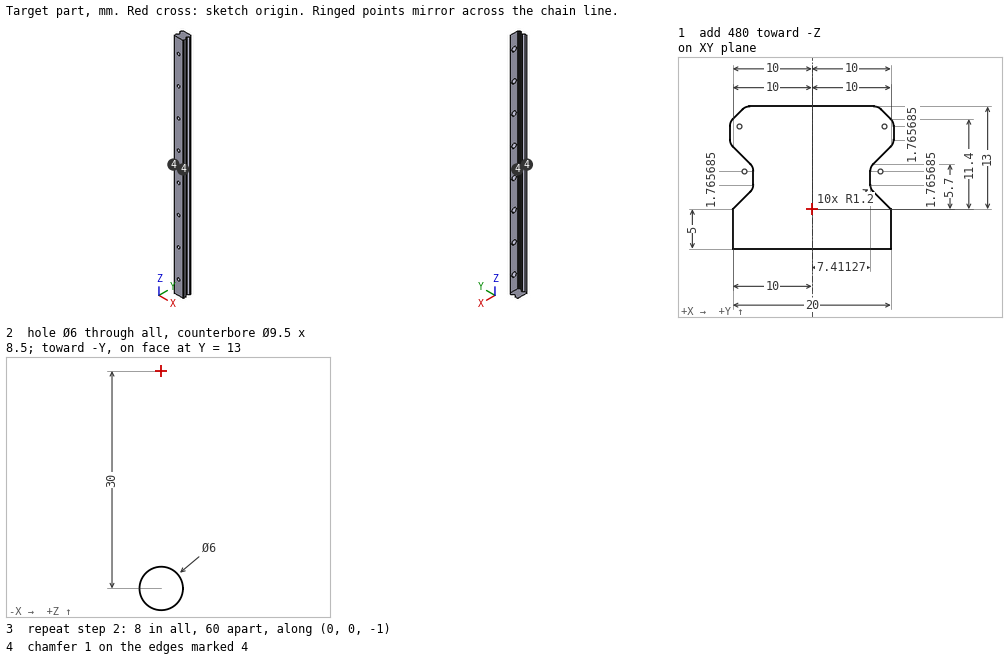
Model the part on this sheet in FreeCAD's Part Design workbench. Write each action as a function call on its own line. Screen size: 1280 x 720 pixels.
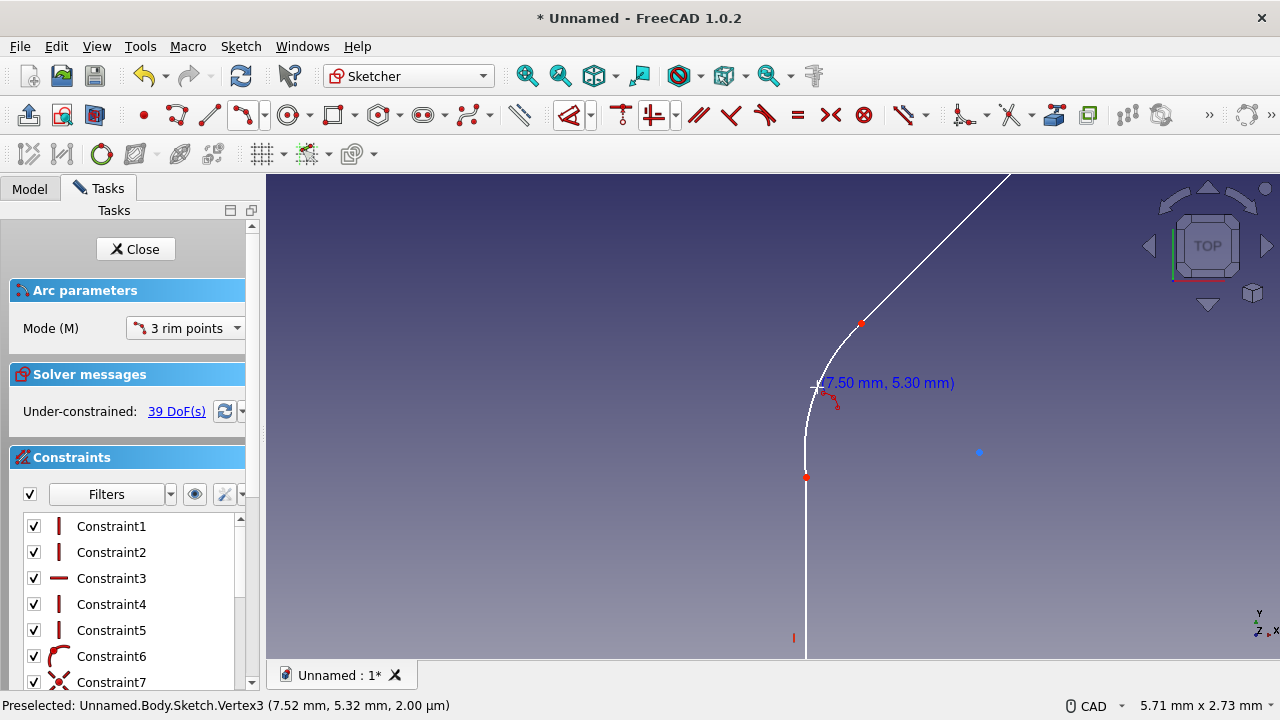
scroll(826, 396, down, 12)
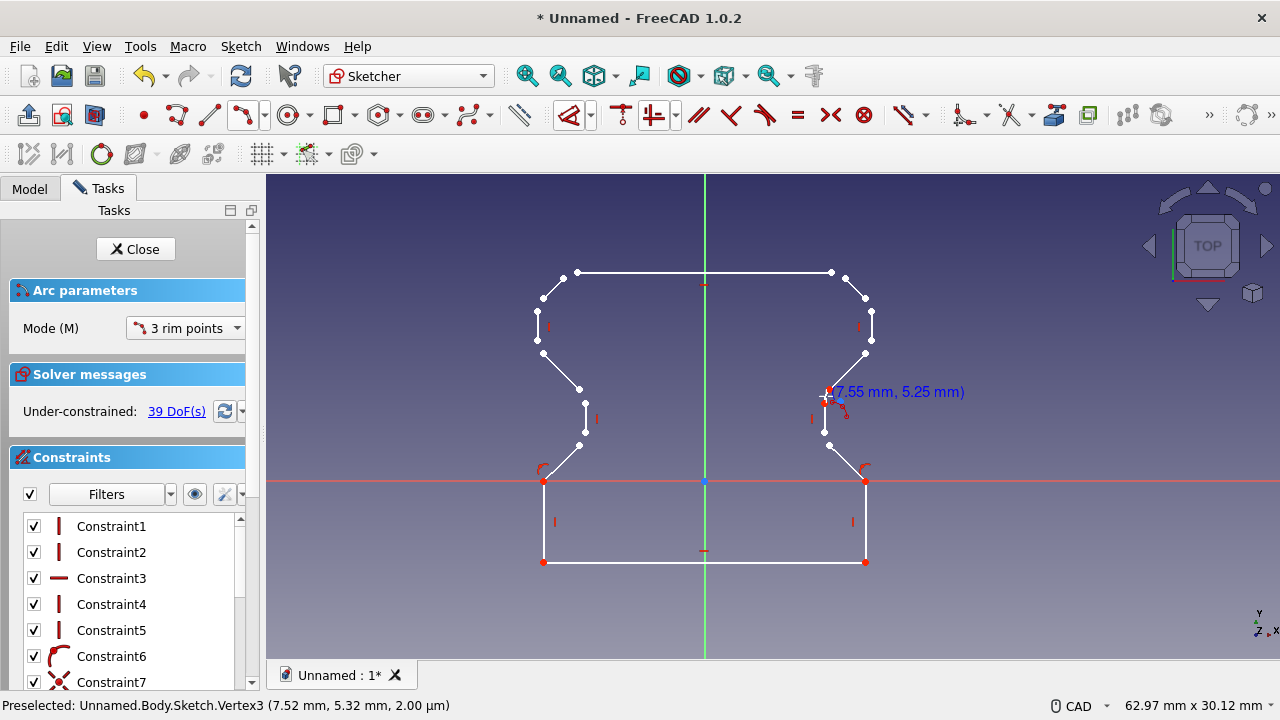
click(866, 354)
click(872, 341)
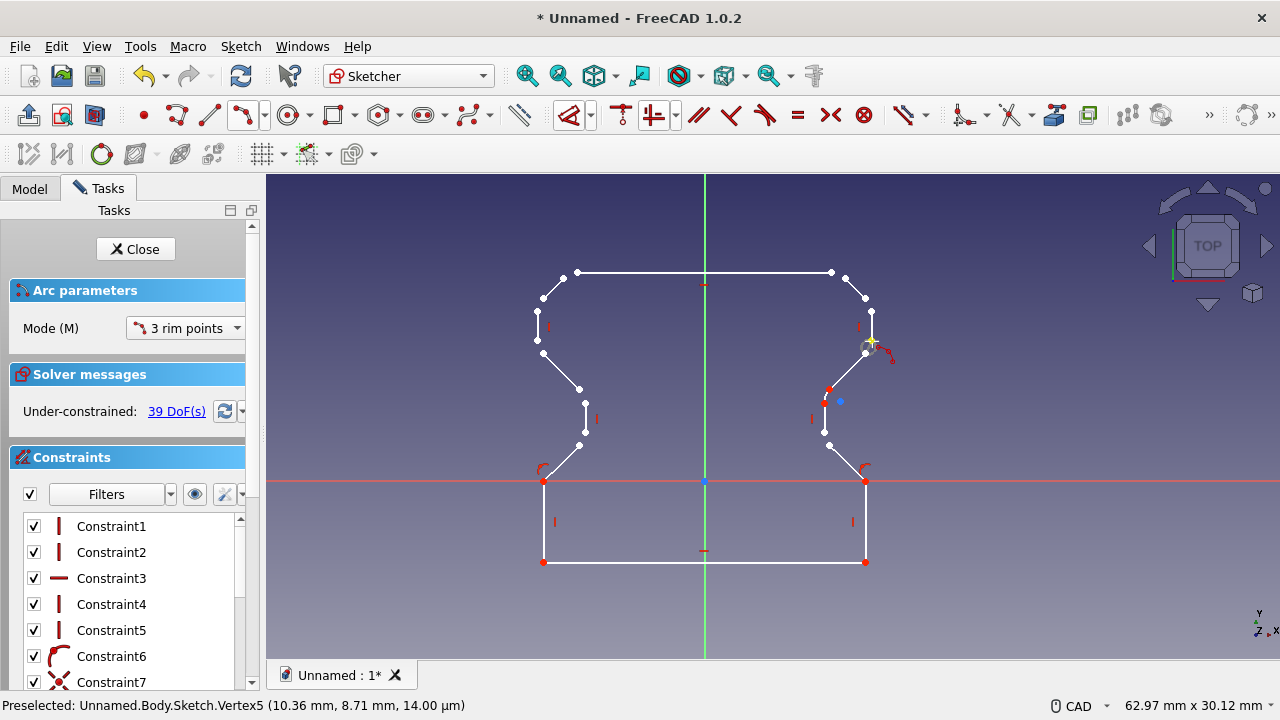
scroll(870, 347, up, 12)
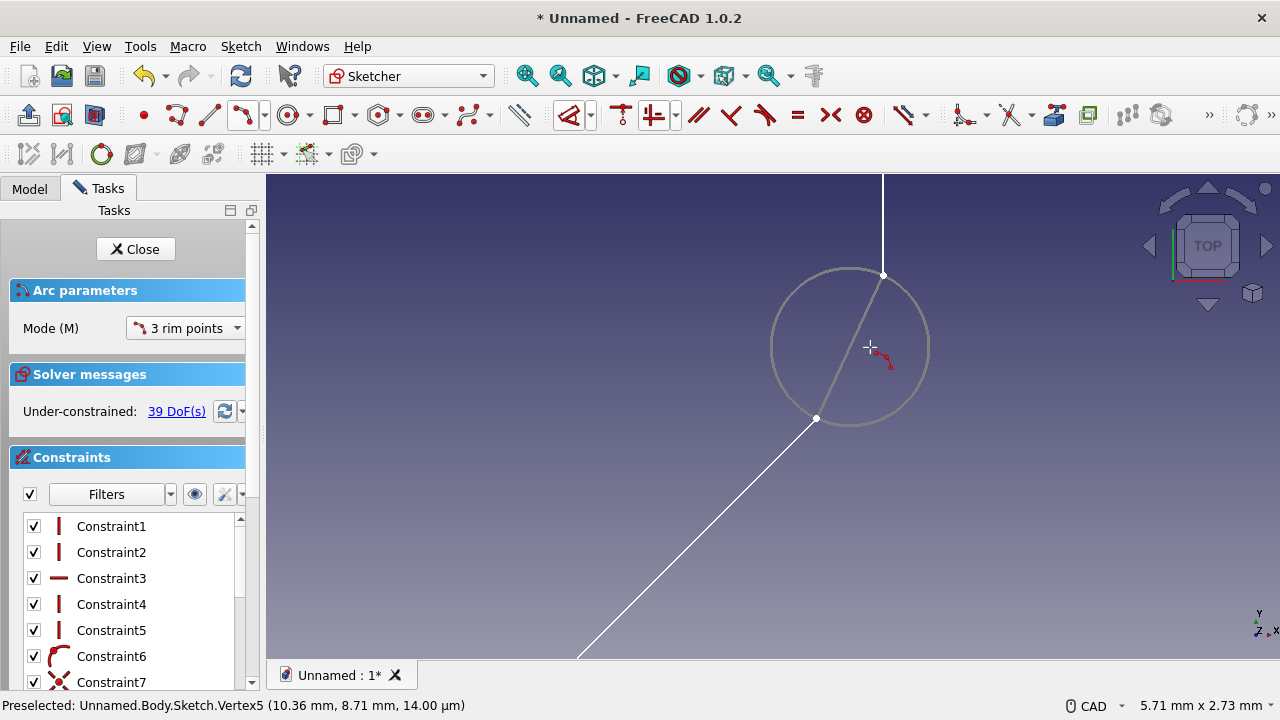
click(865, 344)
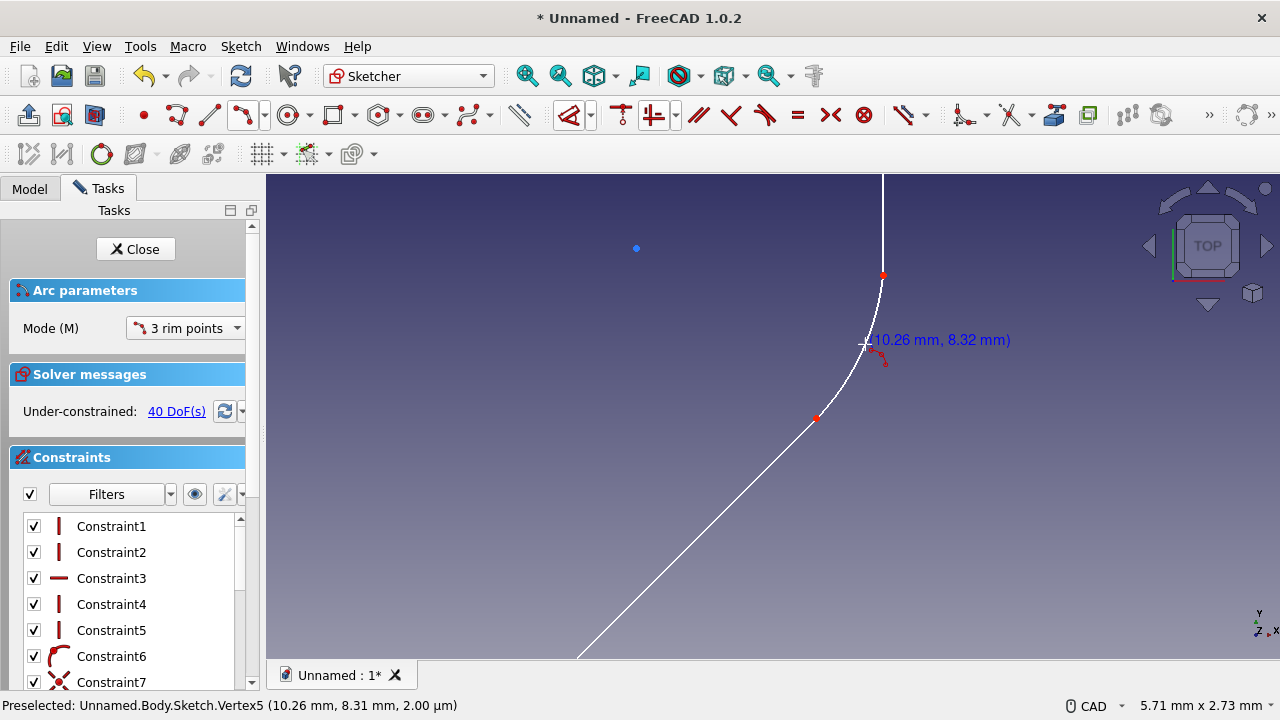
scroll(870, 347, down, 12)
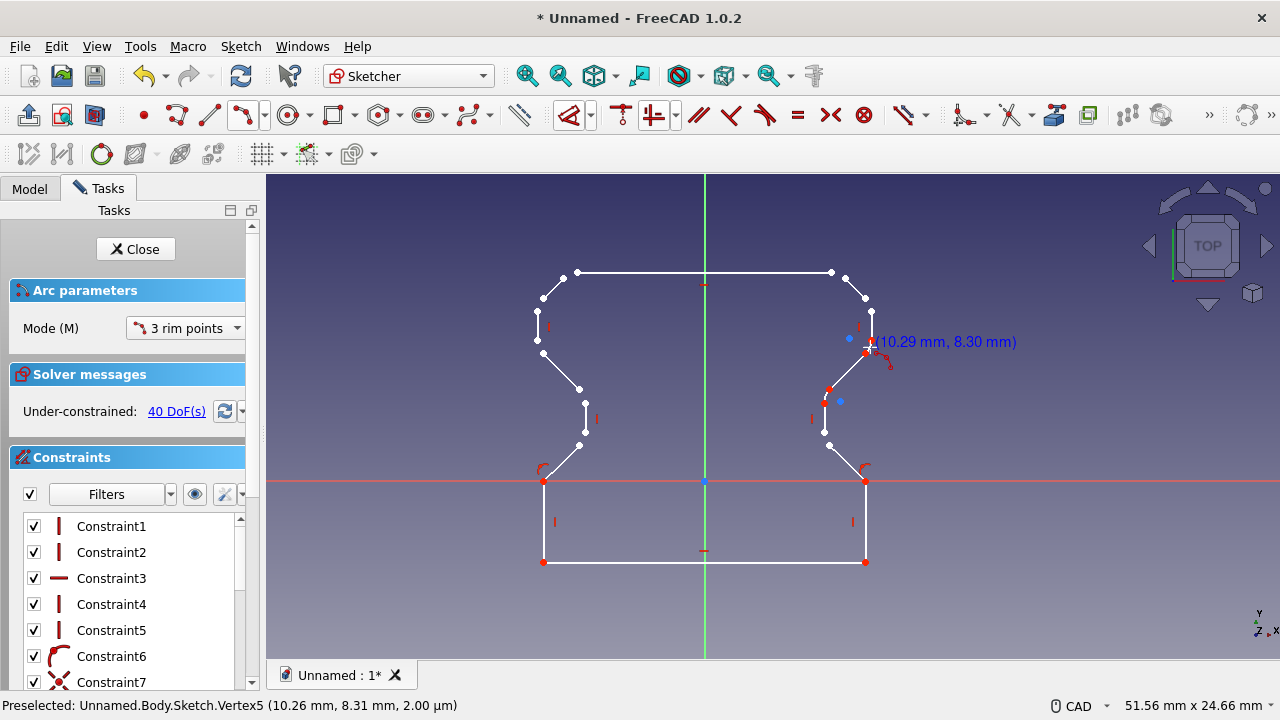
click(872, 312)
click(866, 299)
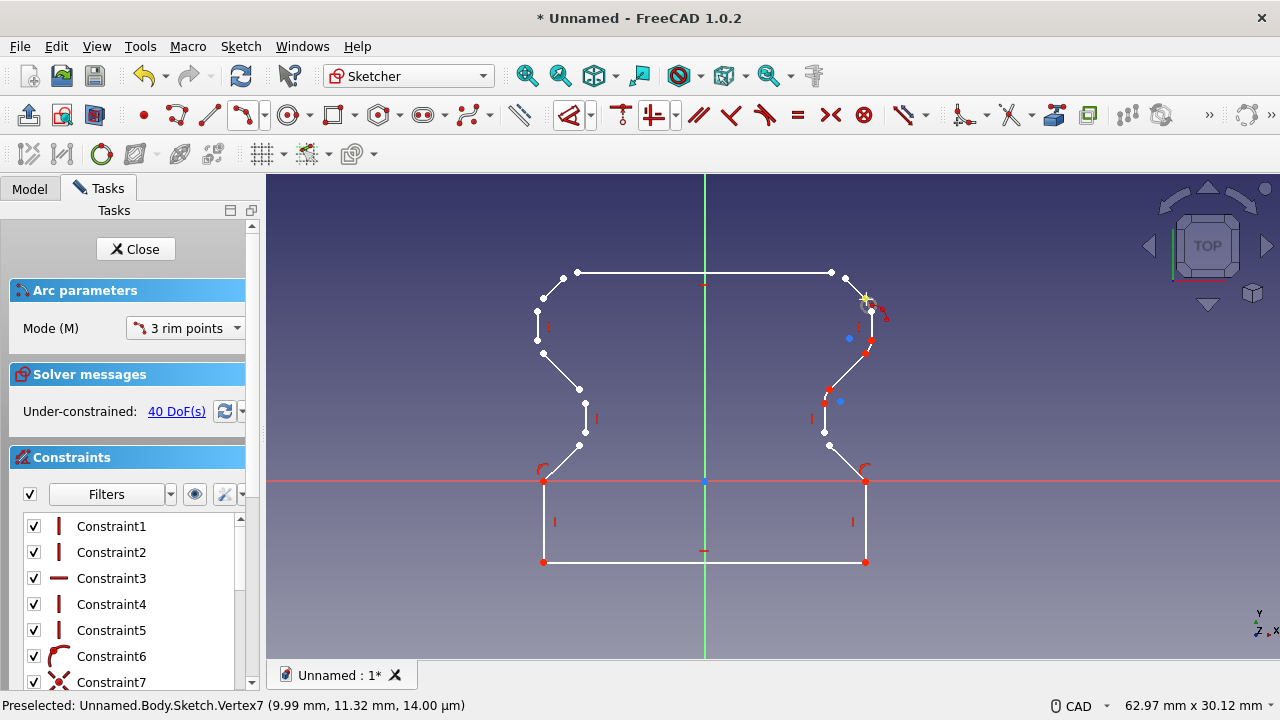
scroll(870, 304, up, 12)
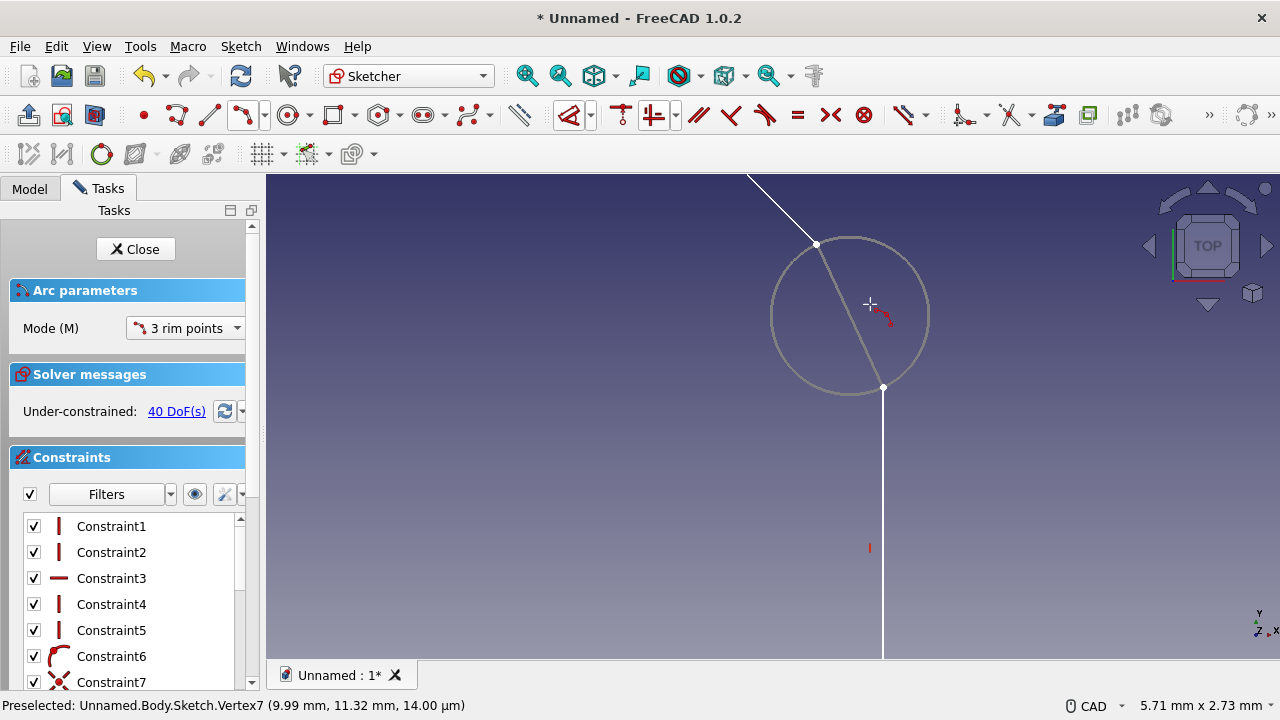
click(865, 299)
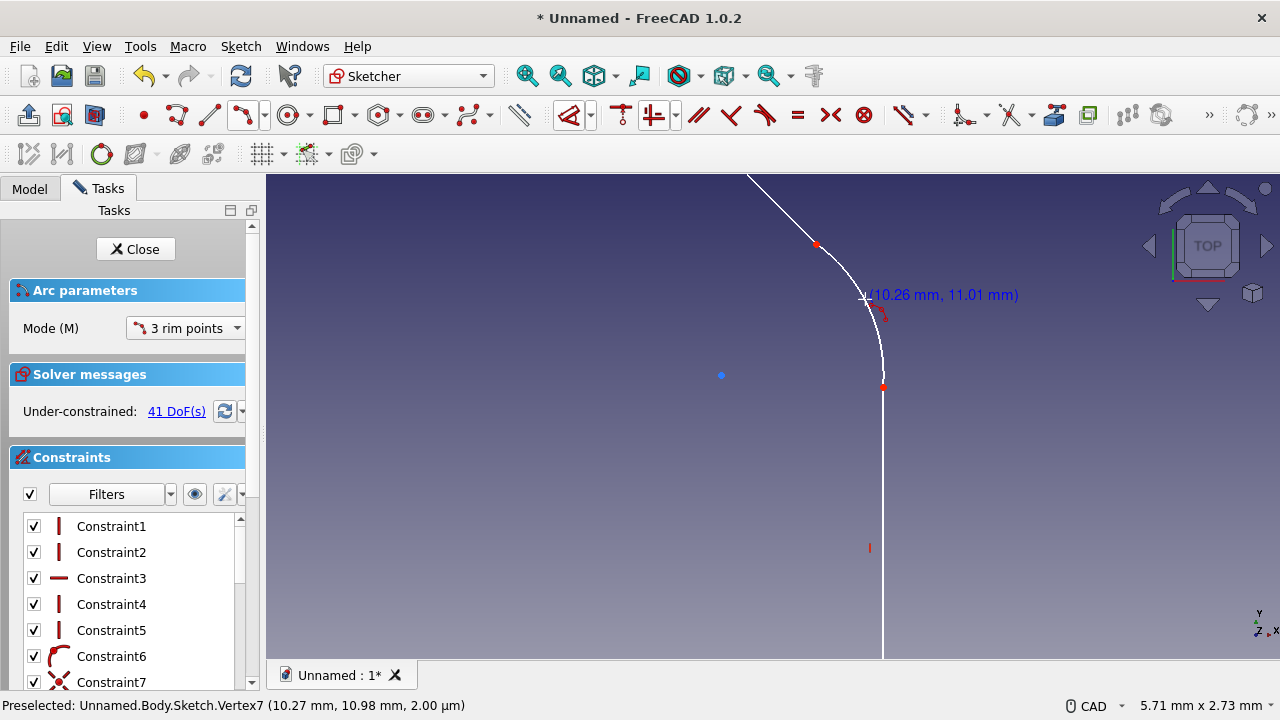
scroll(870, 304, down, 12)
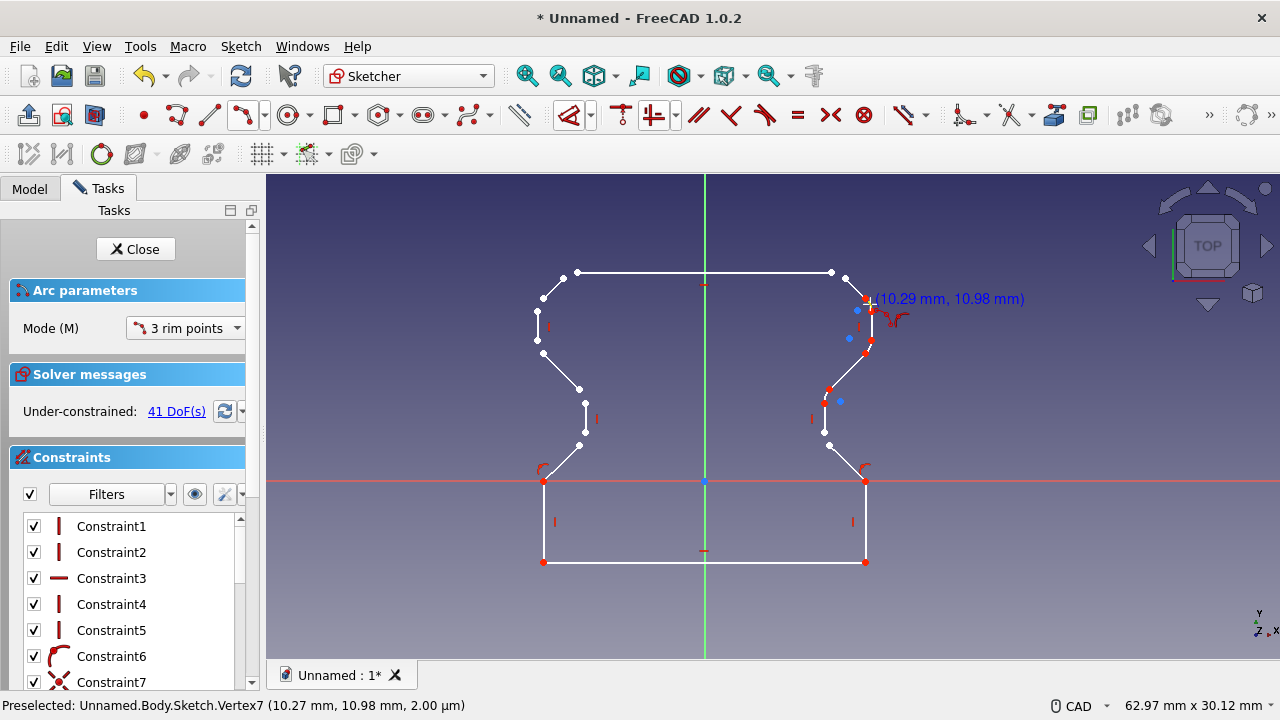
click(846, 279)
click(832, 273)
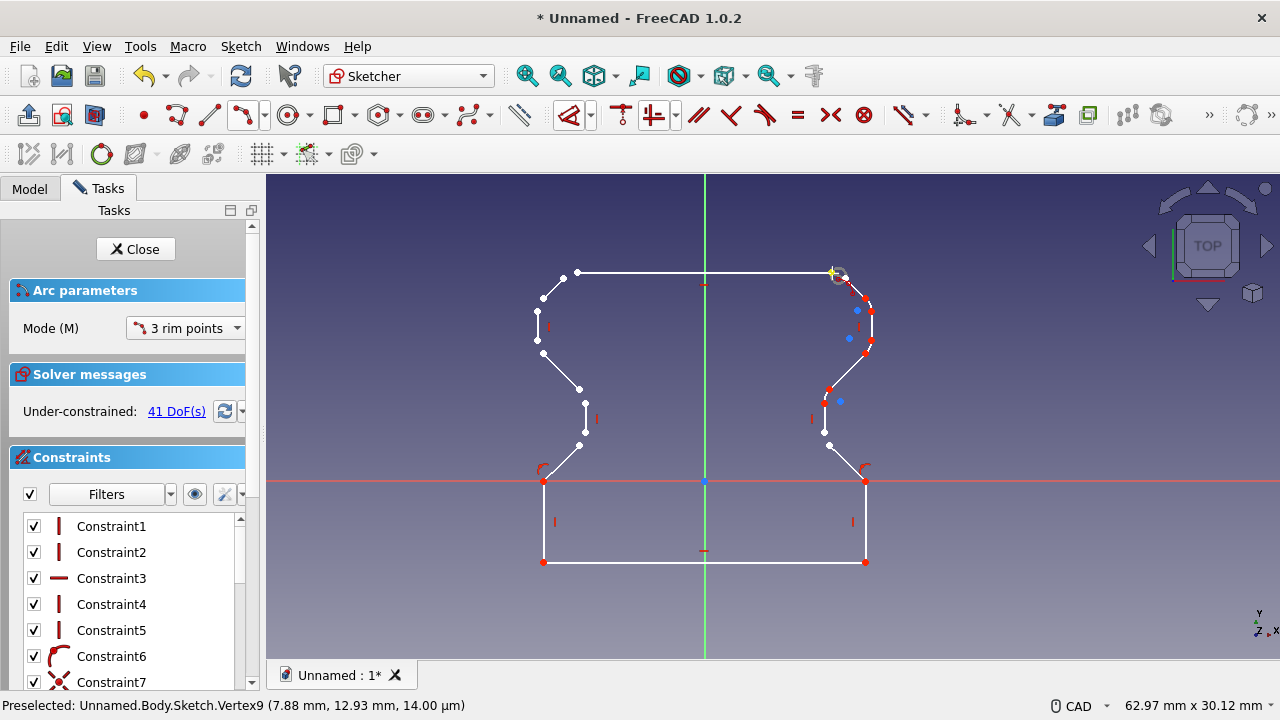
scroll(840, 273, up, 12)